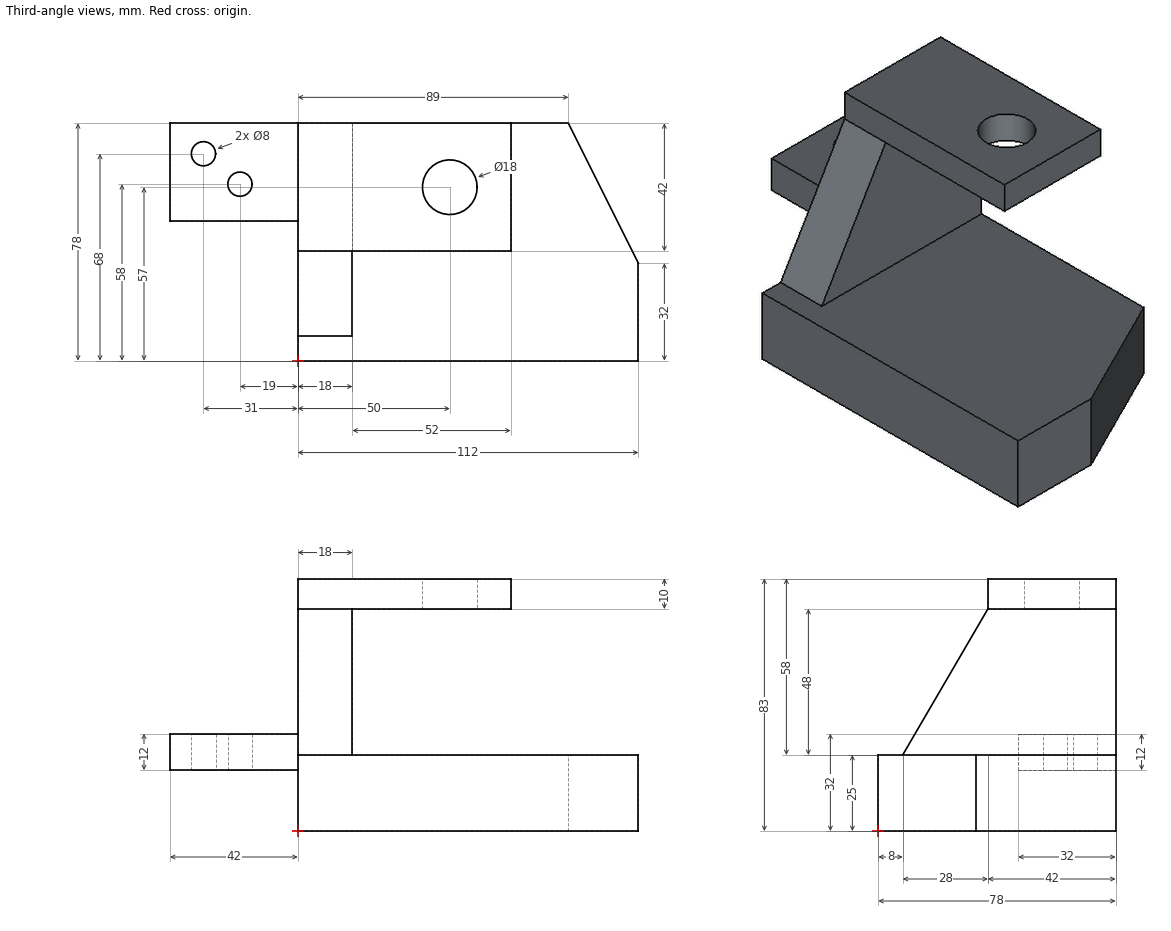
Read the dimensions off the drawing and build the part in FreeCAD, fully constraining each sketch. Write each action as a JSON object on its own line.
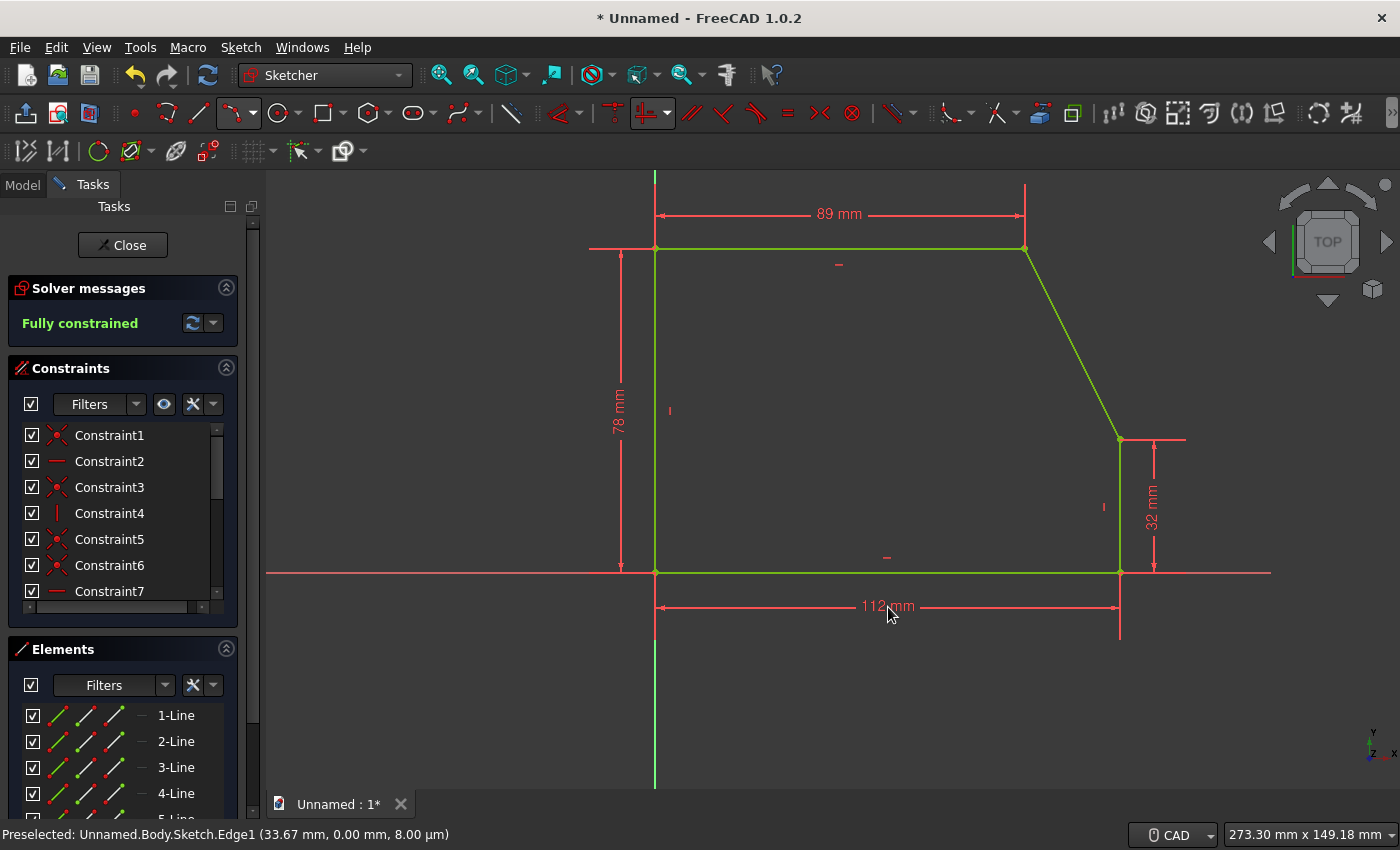
{"action": "left_click", "coordinate": [123, 245]}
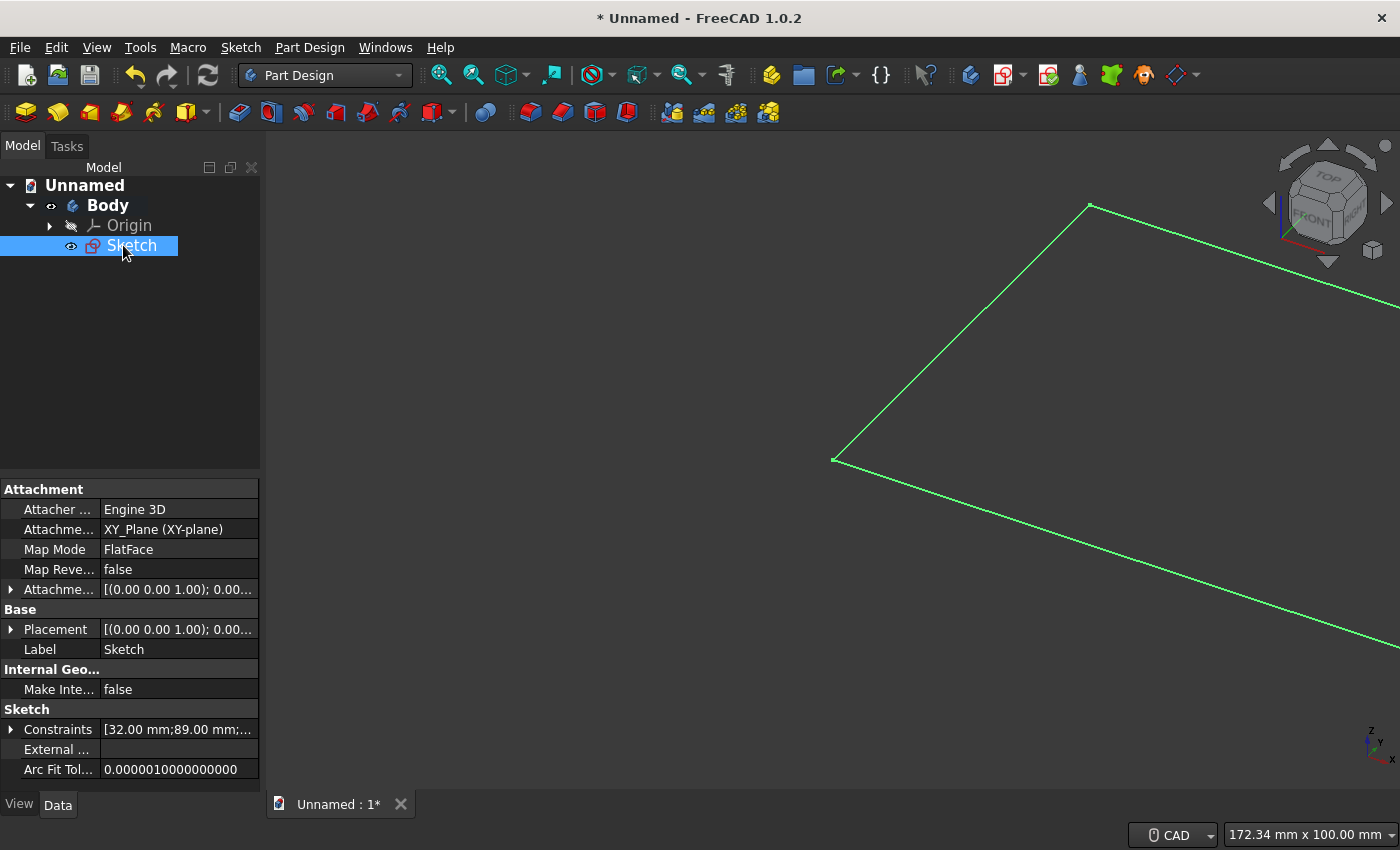
{"action": "left_click", "coordinate": [26, 112]}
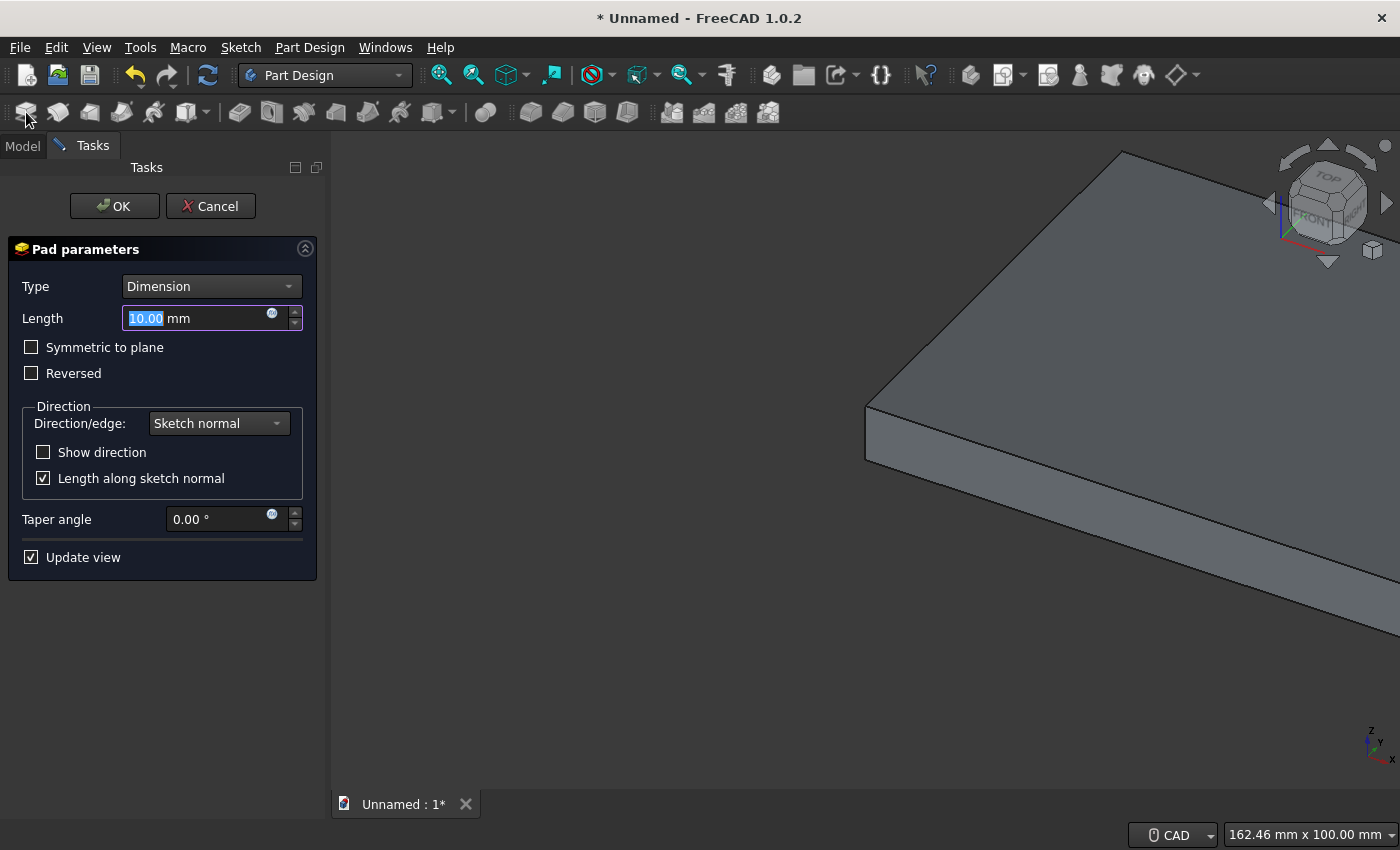
{"action": "type", "text": "25"}
{"action": "key", "text": "Tab"}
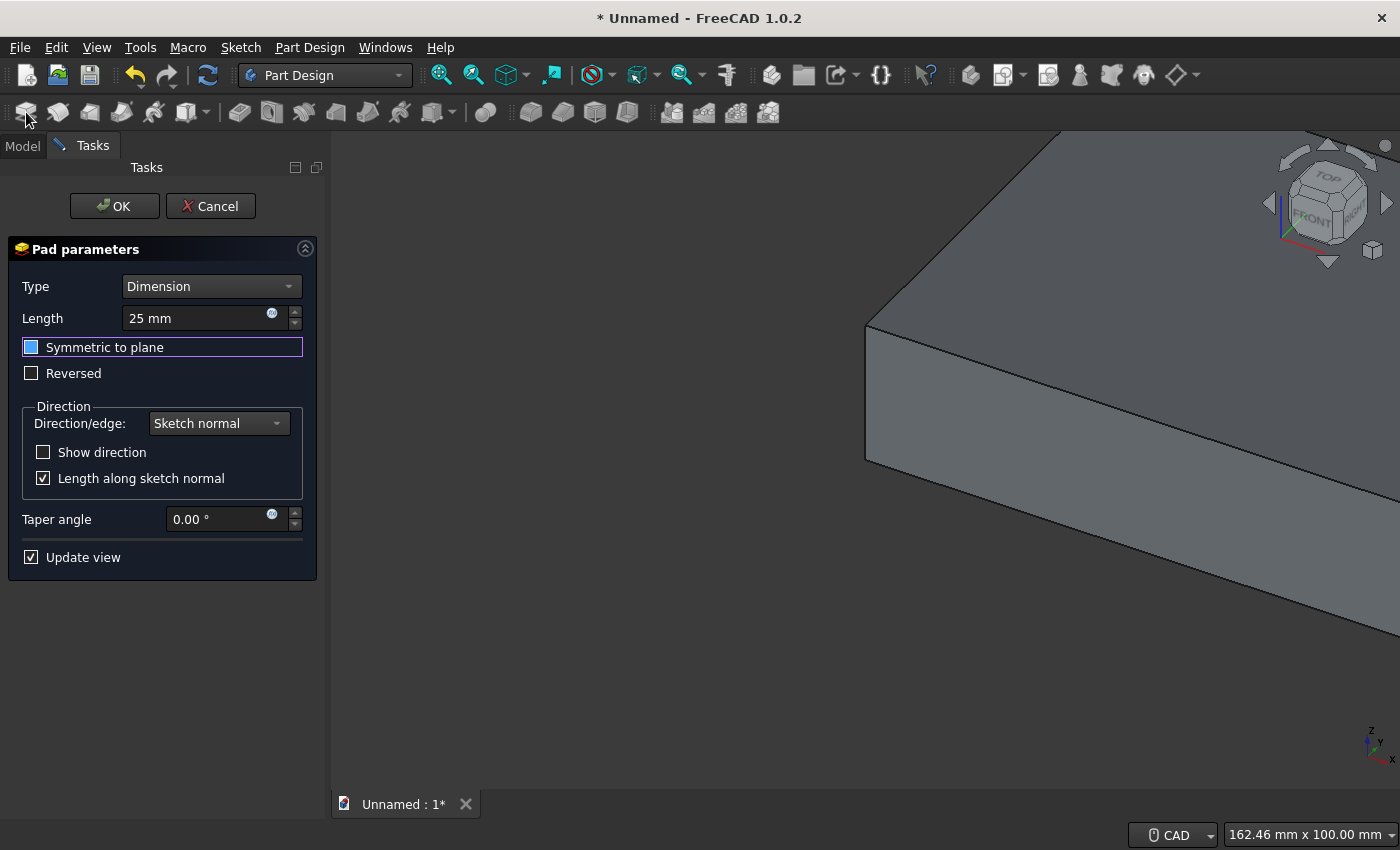
{"action": "left_click", "coordinate": [115, 206]}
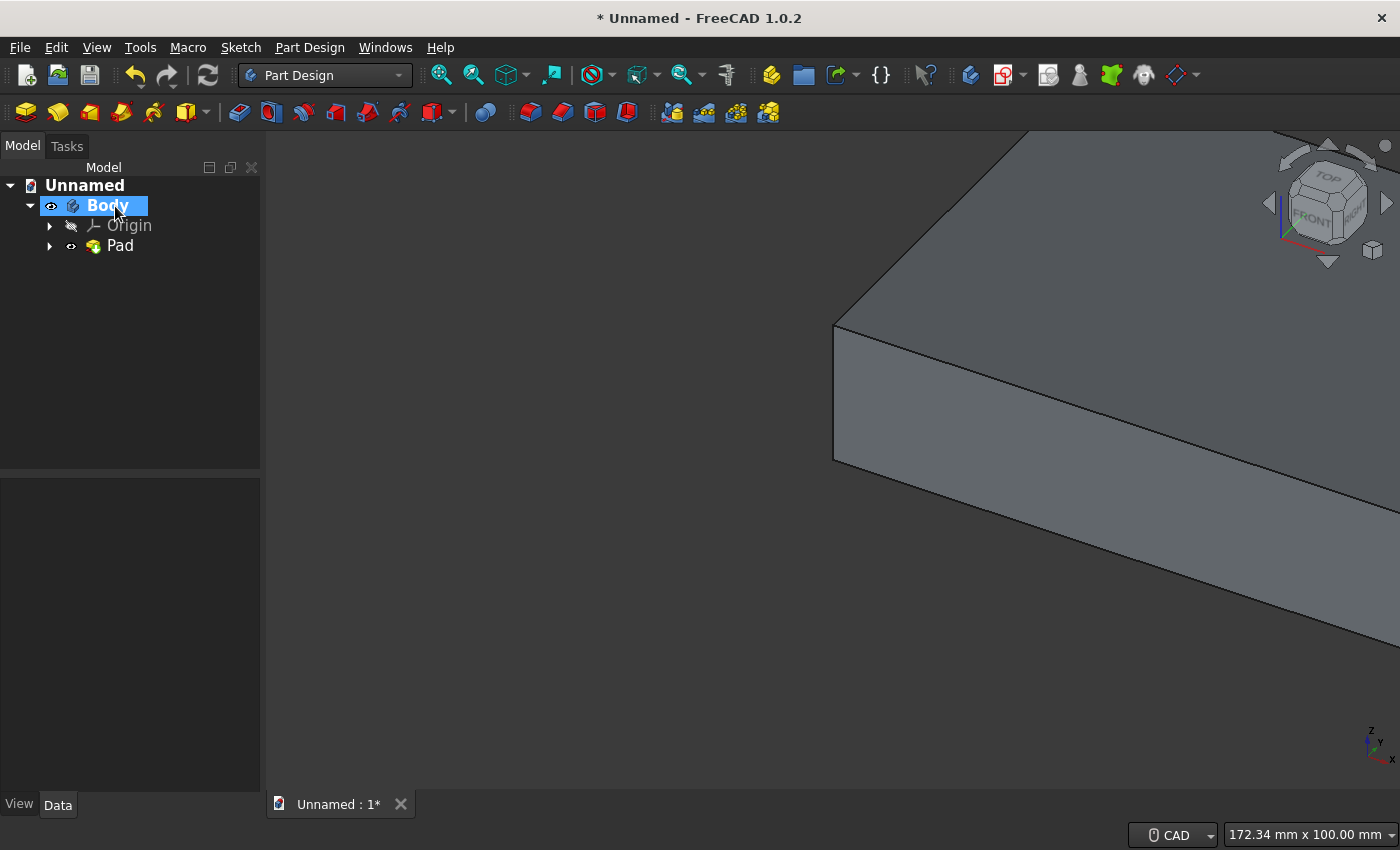
{"action": "key", "text": "v f"}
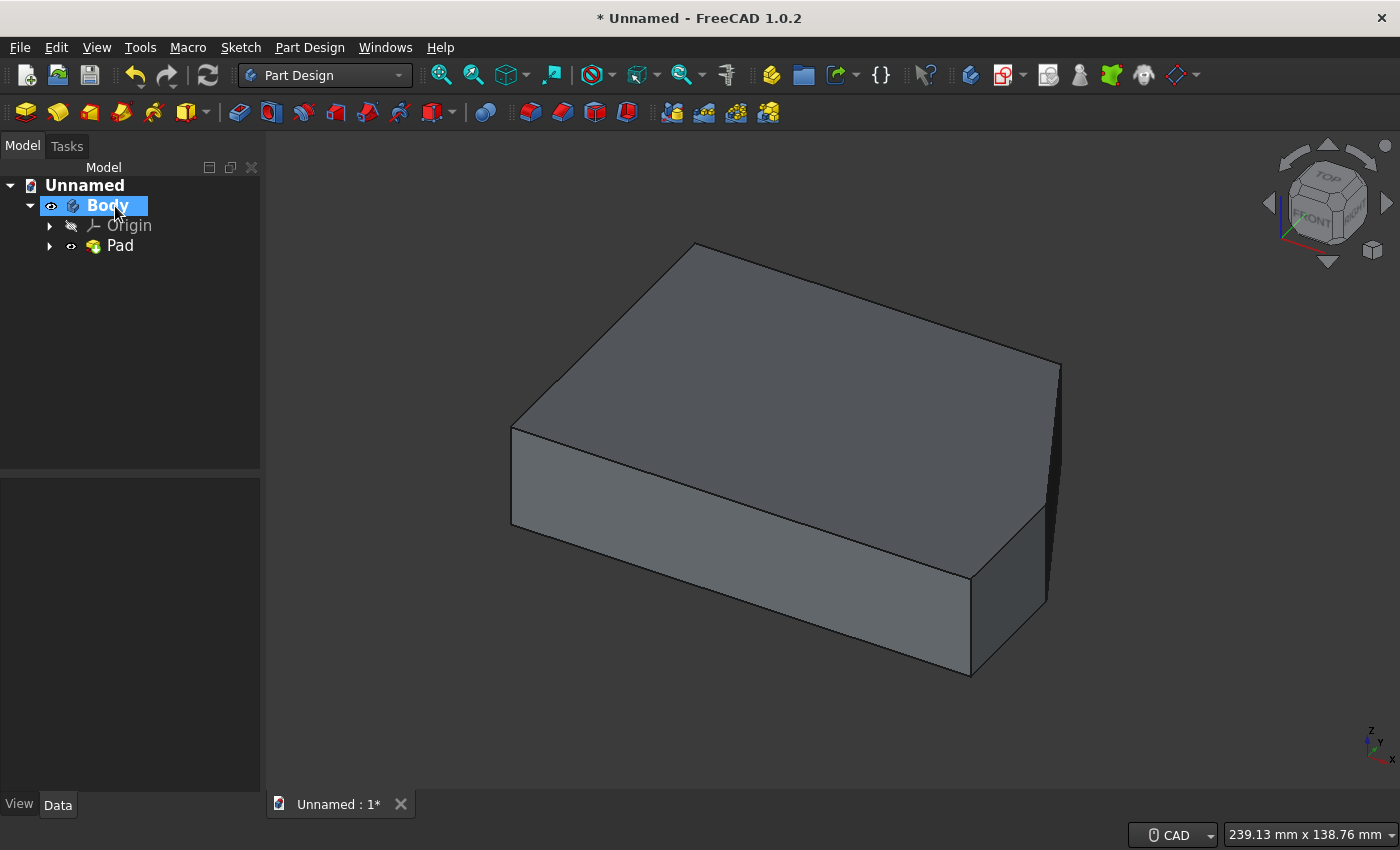
{"action": "key", "text": "6"}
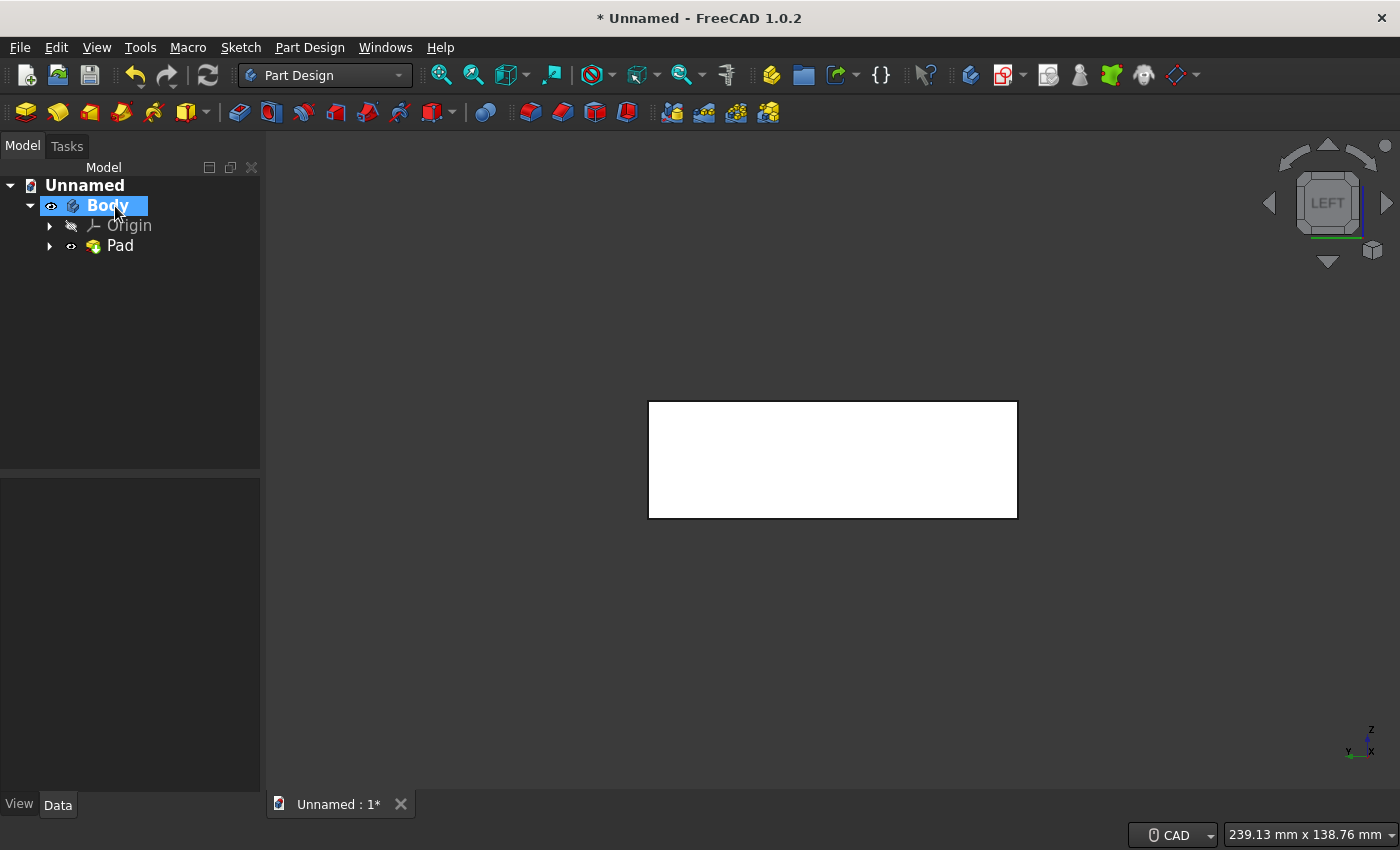
{"action": "left_click", "coordinate": [442, 76]}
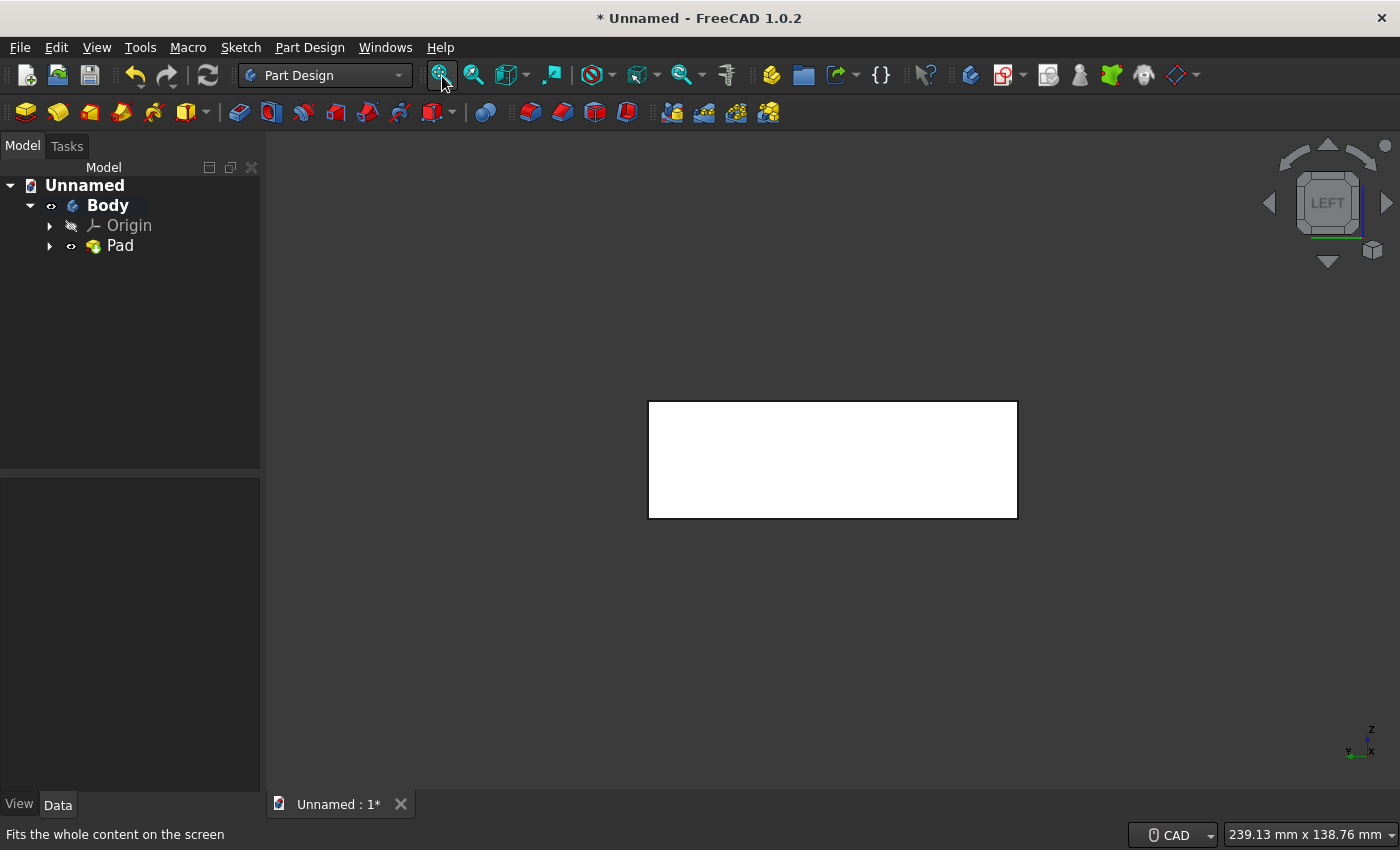
{"action": "left_click", "coordinate": [727, 459]}